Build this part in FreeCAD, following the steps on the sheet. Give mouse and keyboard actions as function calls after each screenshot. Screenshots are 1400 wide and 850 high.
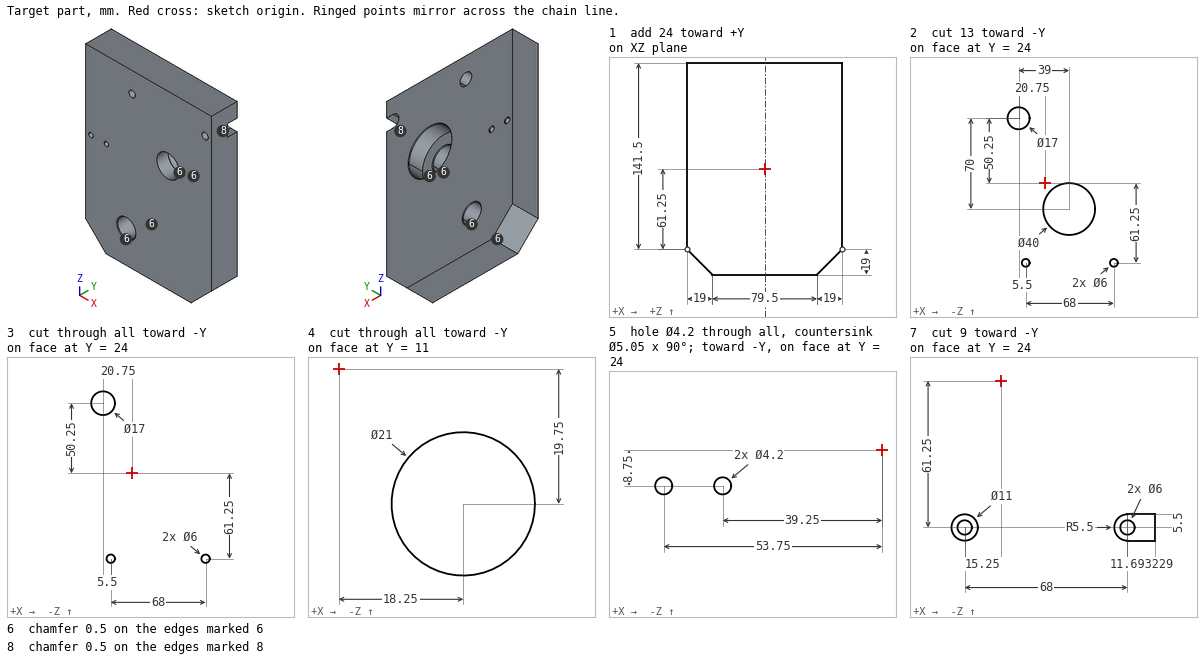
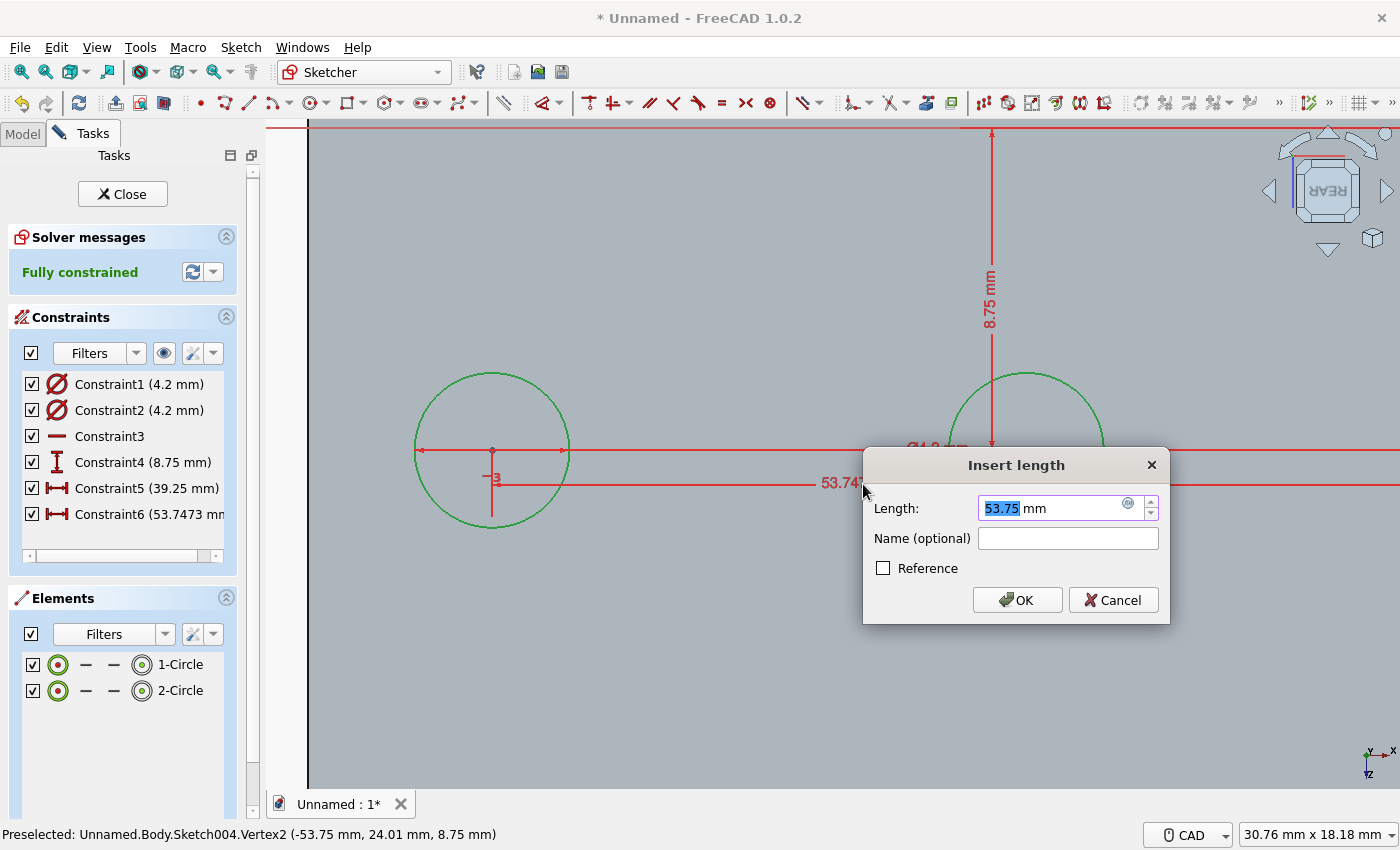
text(53.75)
key(Return)
key(Escape)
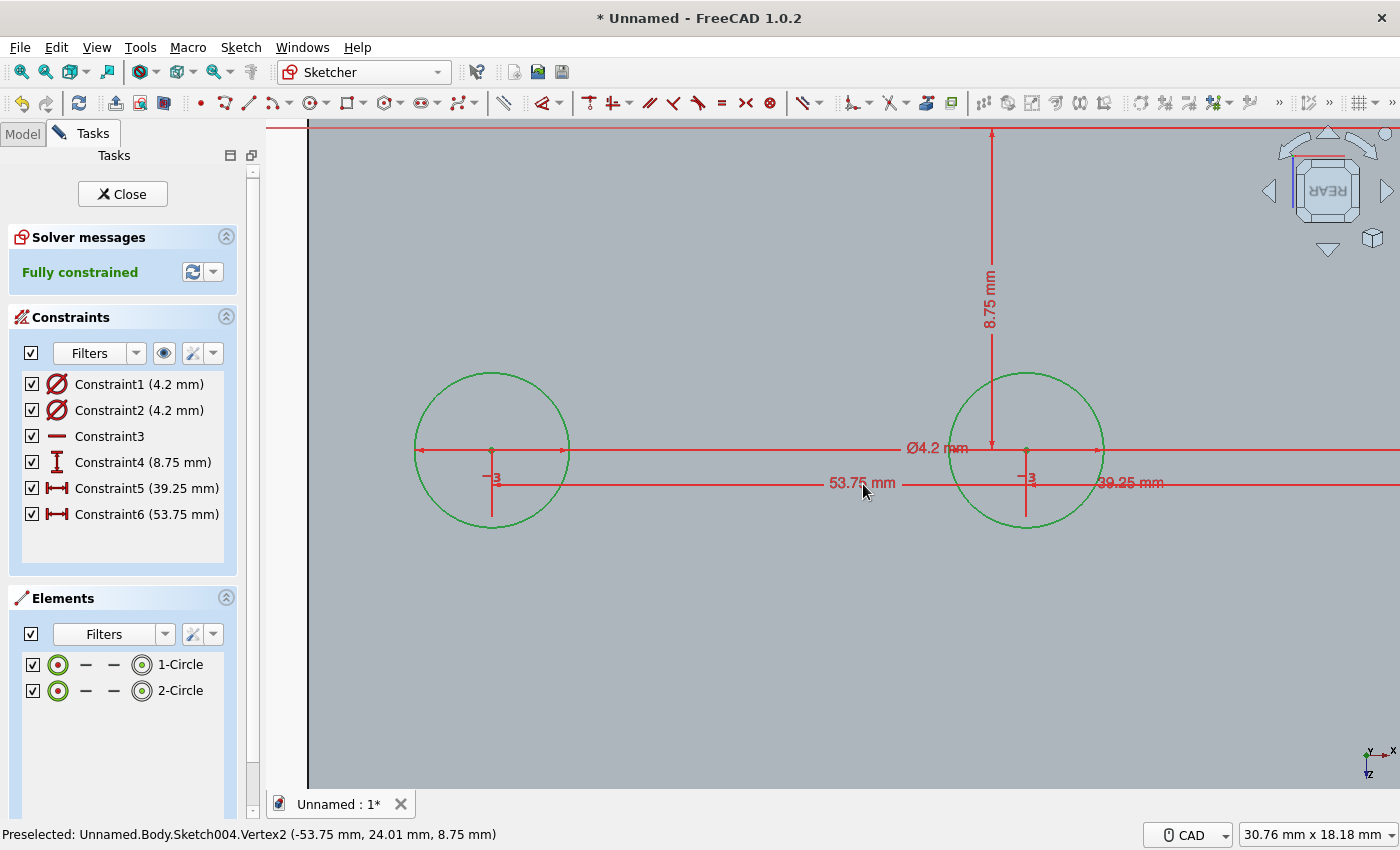
click(123, 194)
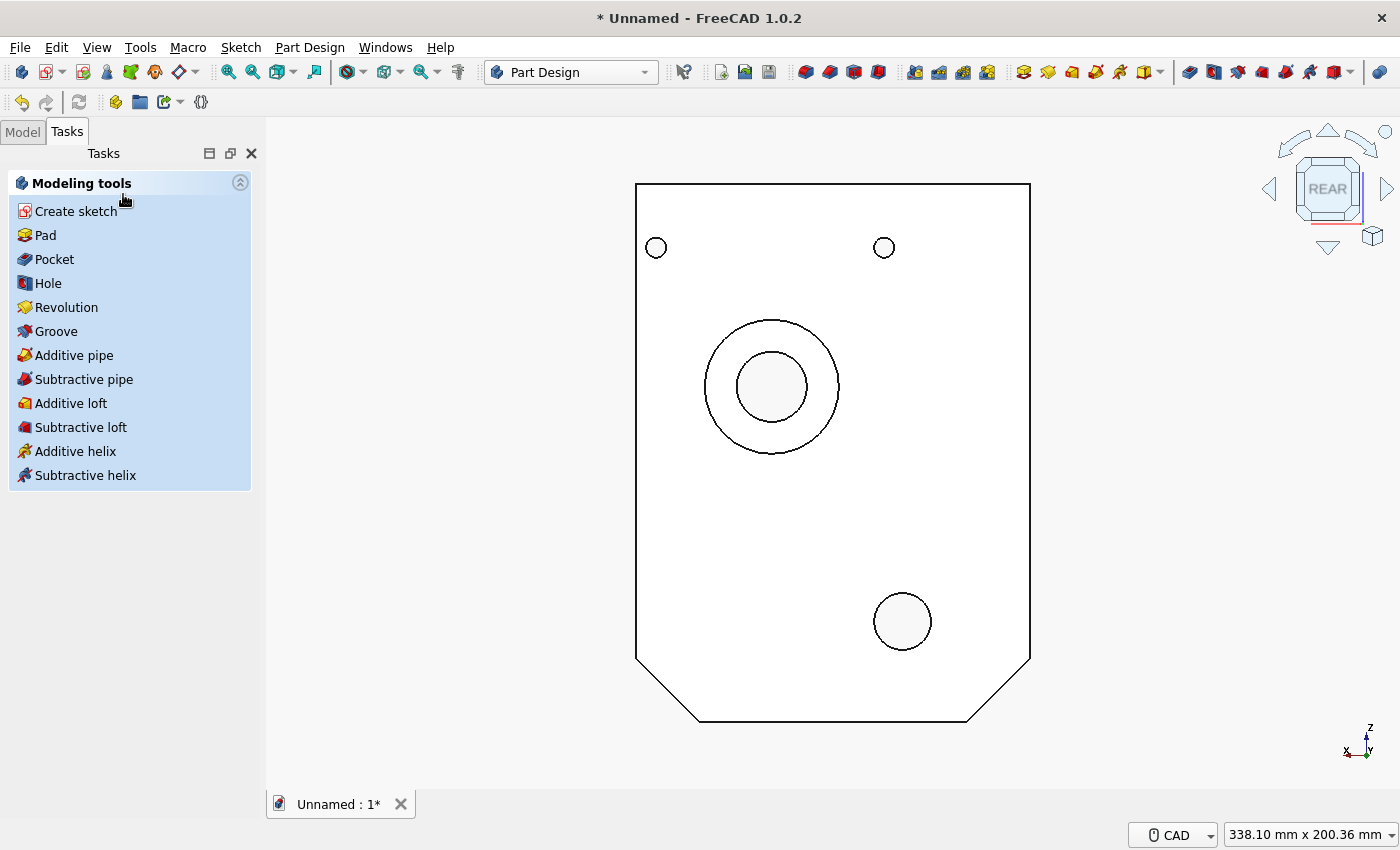
click(1214, 72)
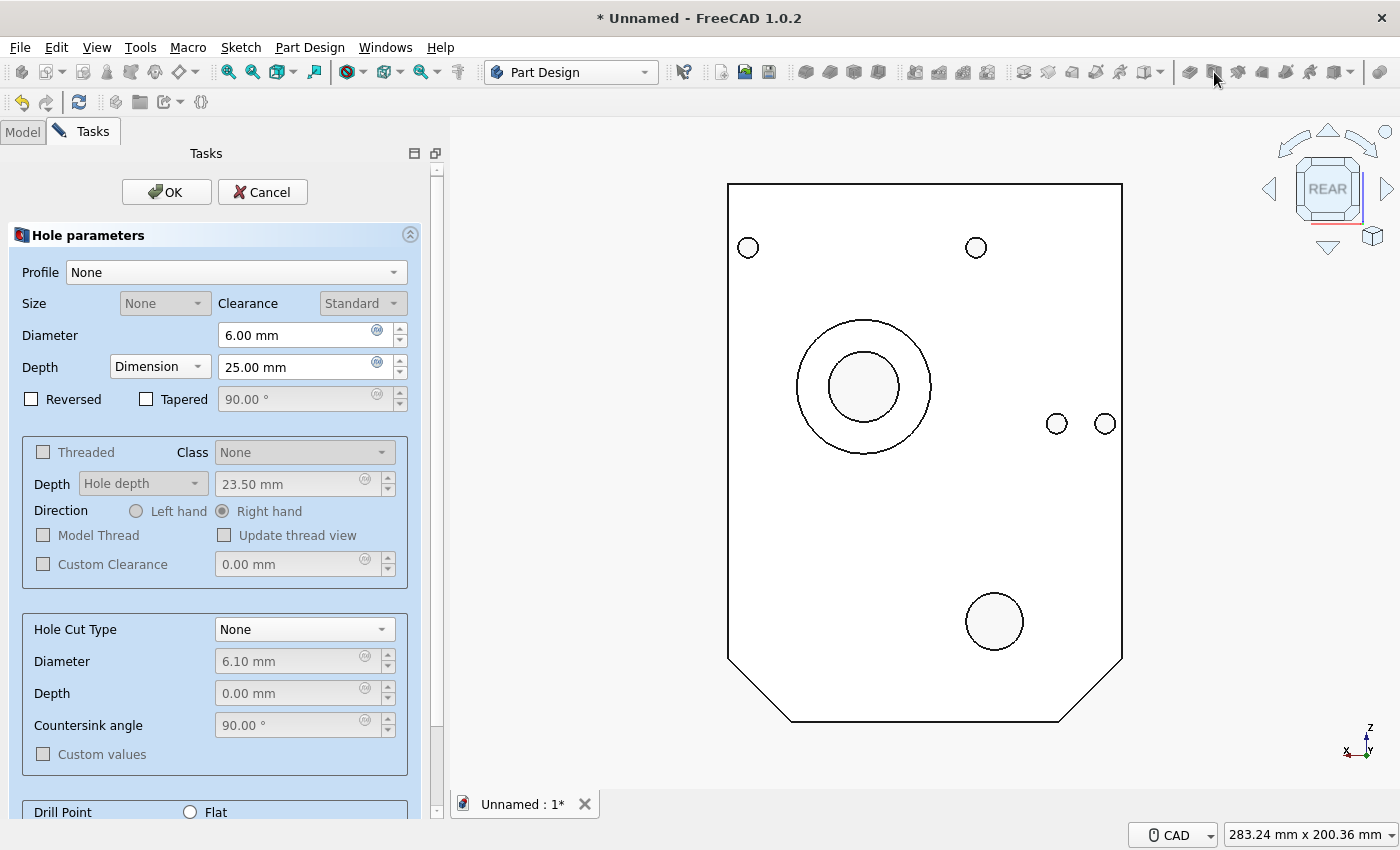
triple_click(305, 335)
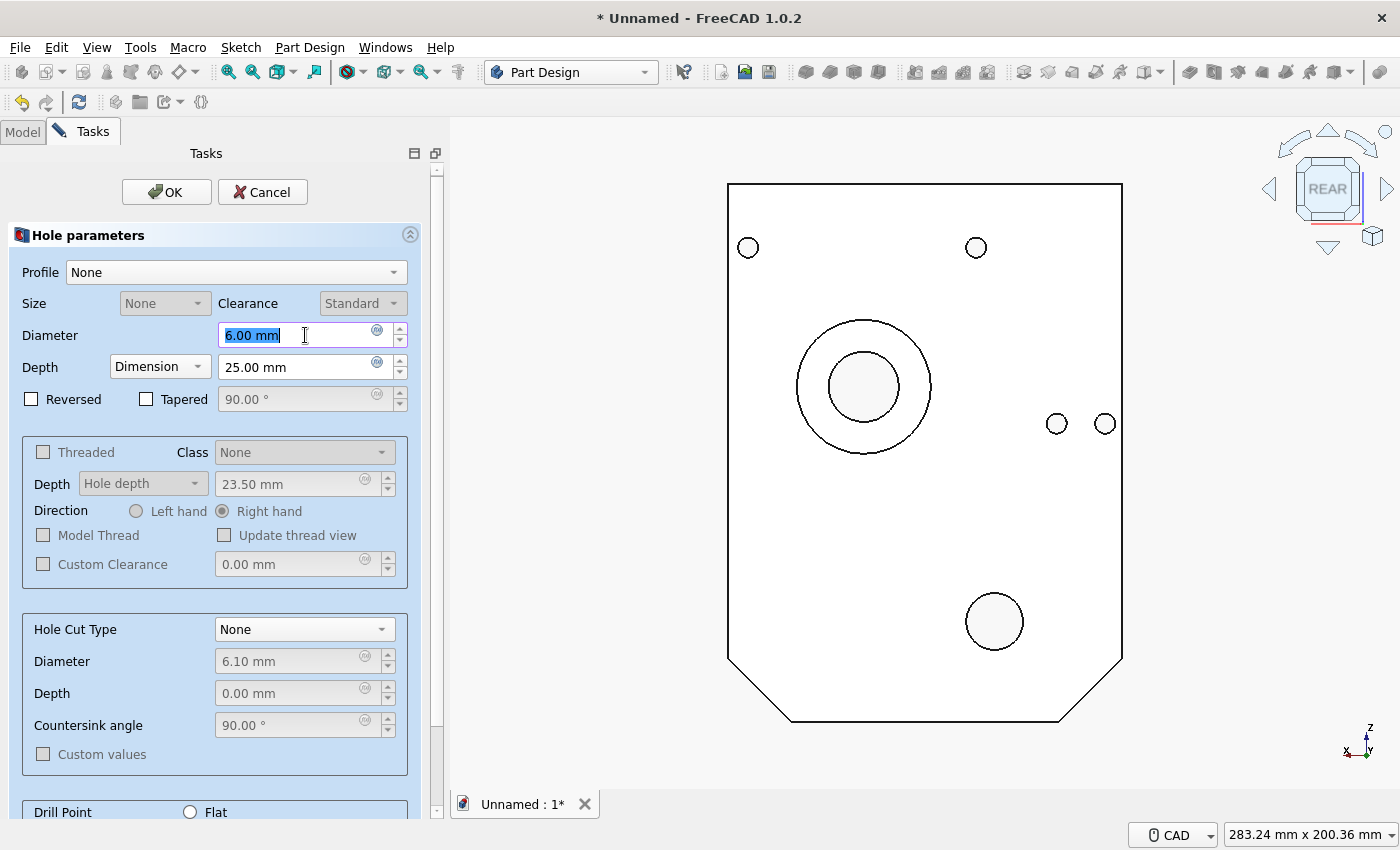
text(4.2)
key(Tab)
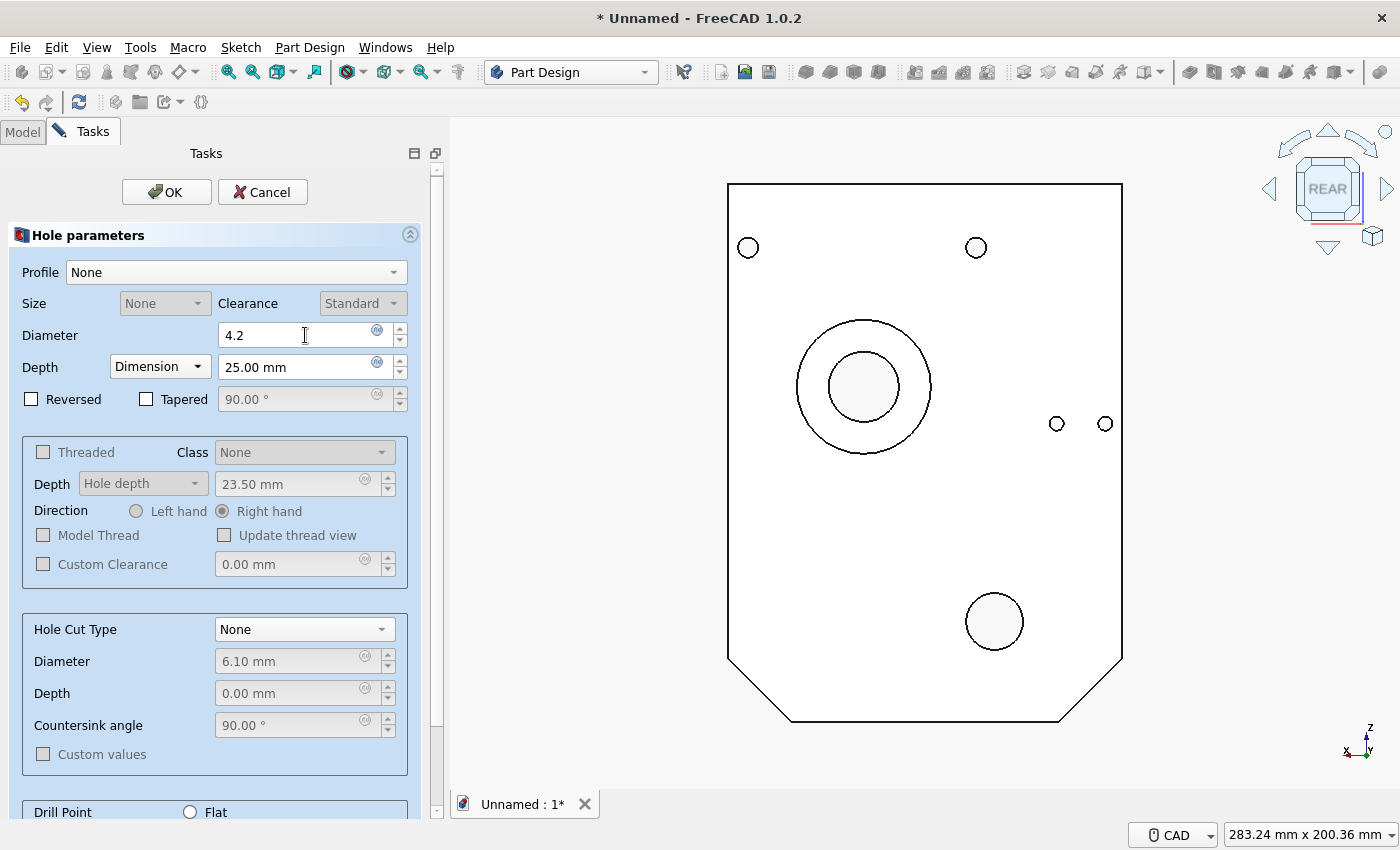
click(161, 366)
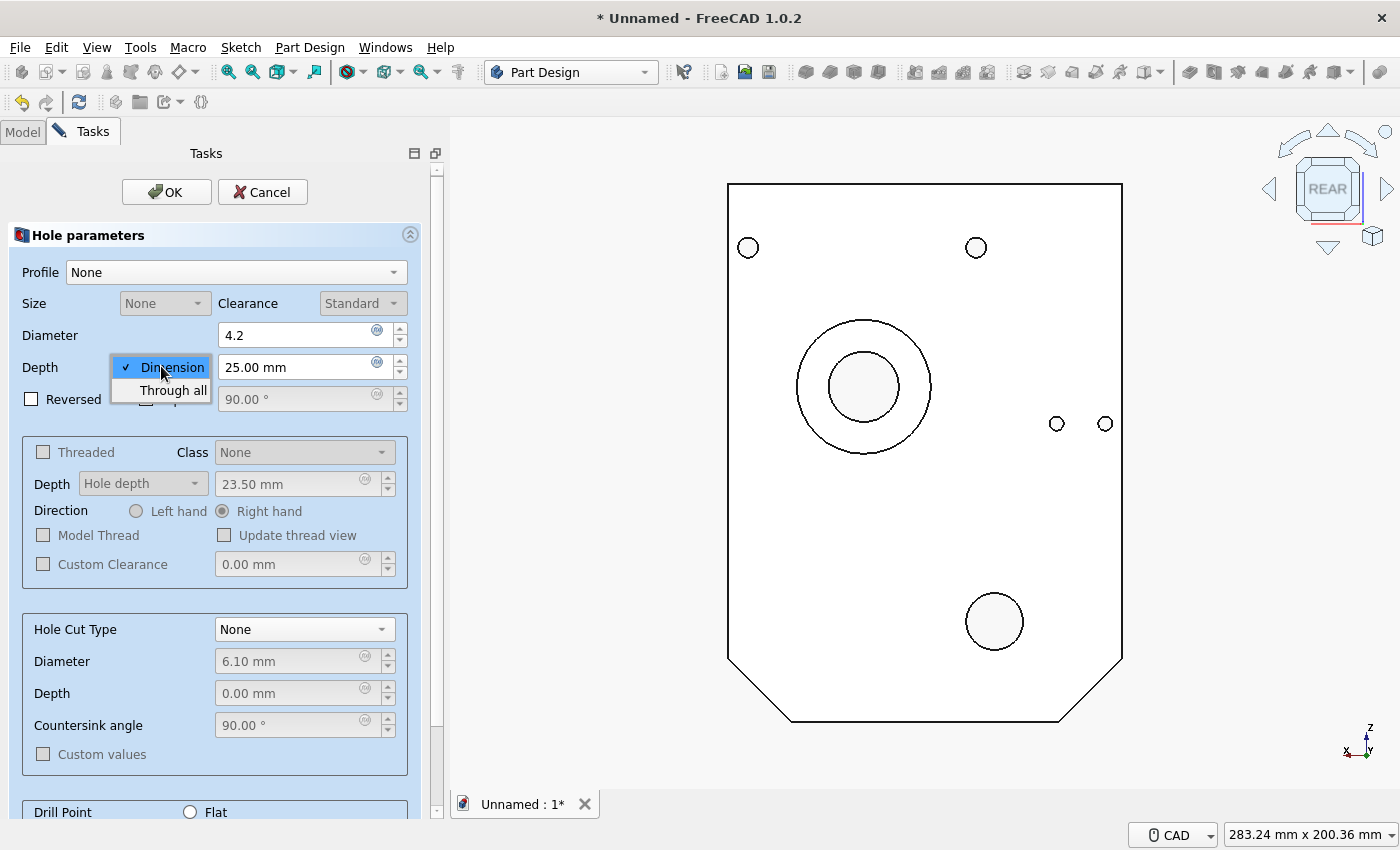
click(160, 390)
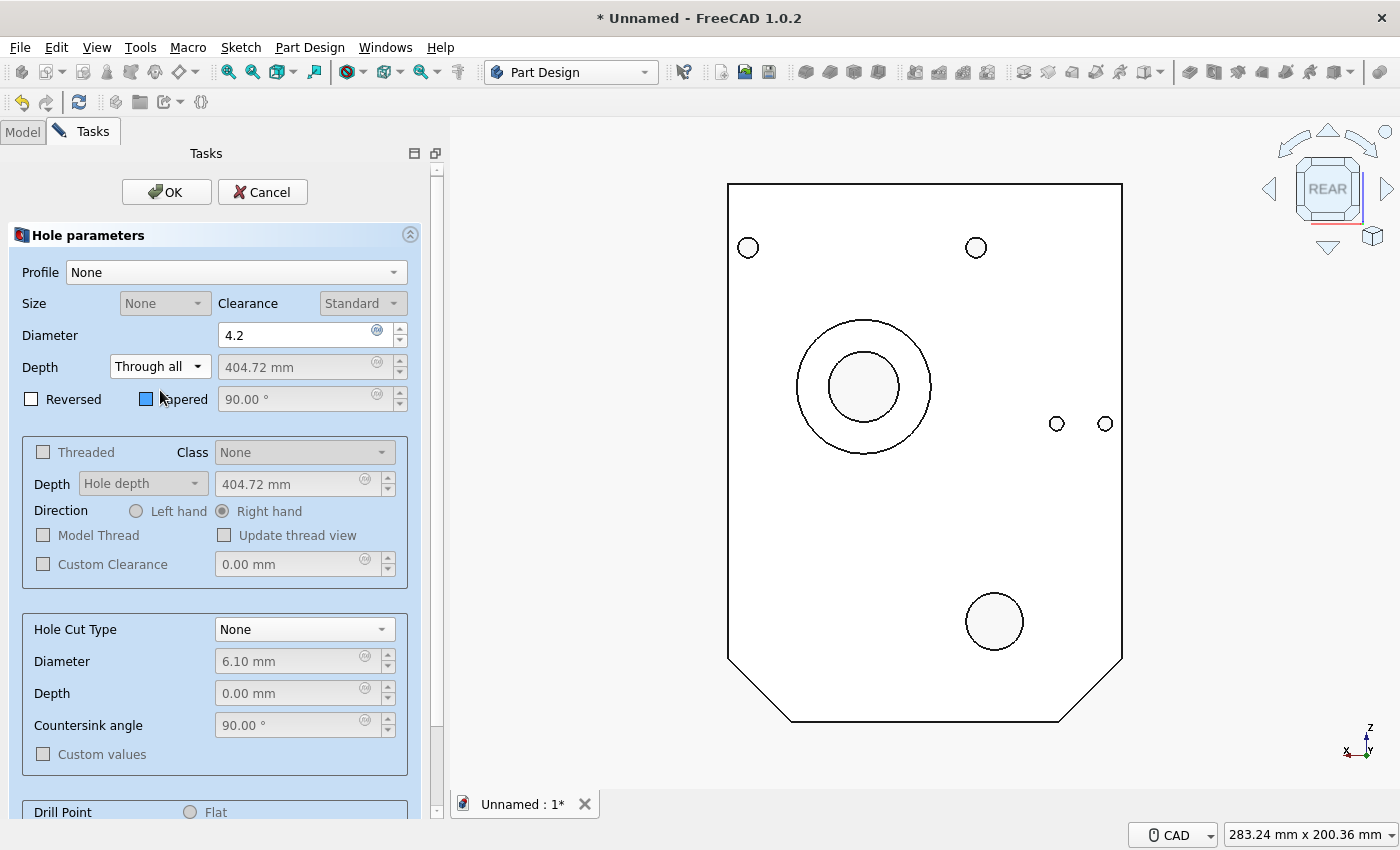
click(306, 630)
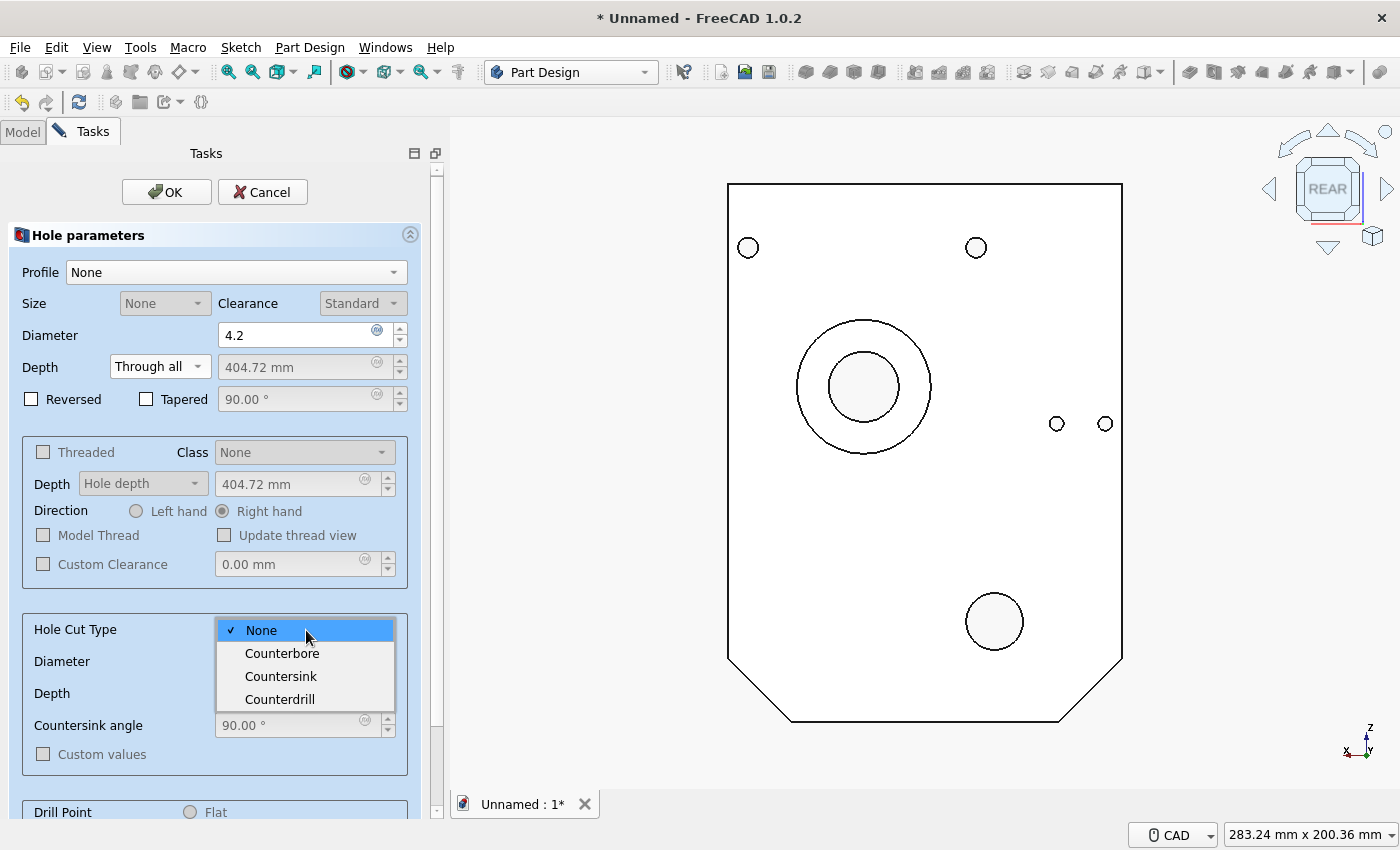
click(304, 676)